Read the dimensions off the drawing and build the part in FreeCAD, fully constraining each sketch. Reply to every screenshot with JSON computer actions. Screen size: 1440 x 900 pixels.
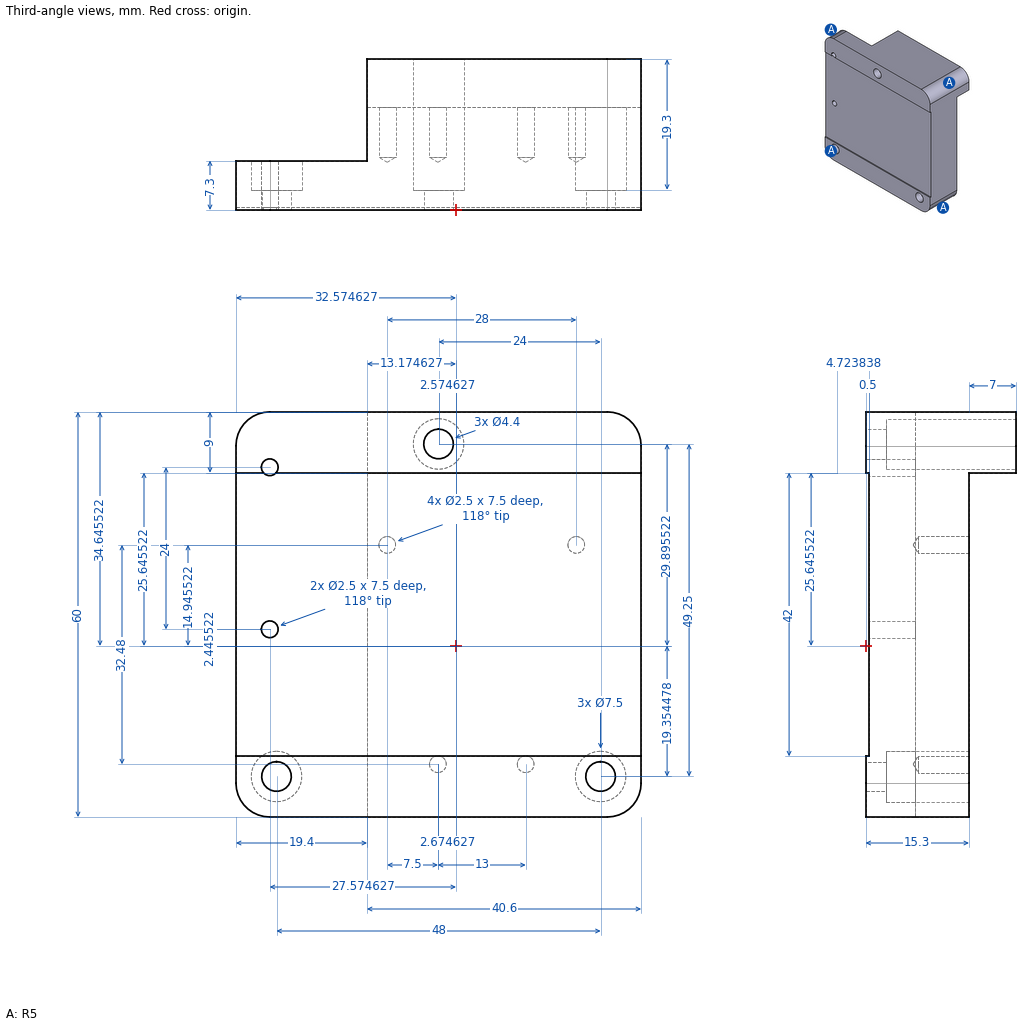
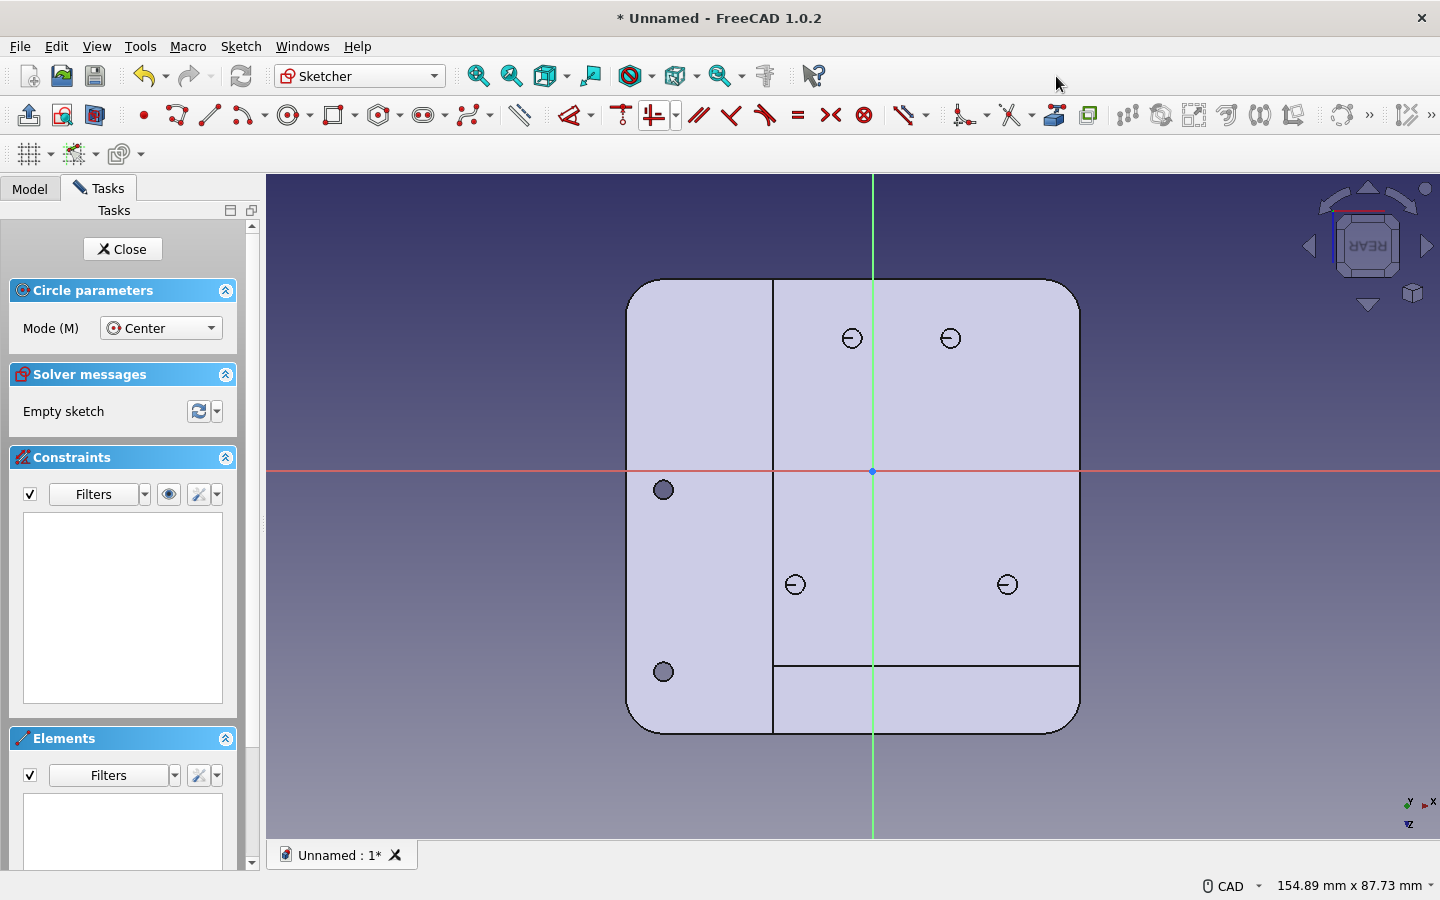
{"action": "left_click", "coordinate": [1035, 325]}
{"action": "left_click", "coordinate": [1055, 304]}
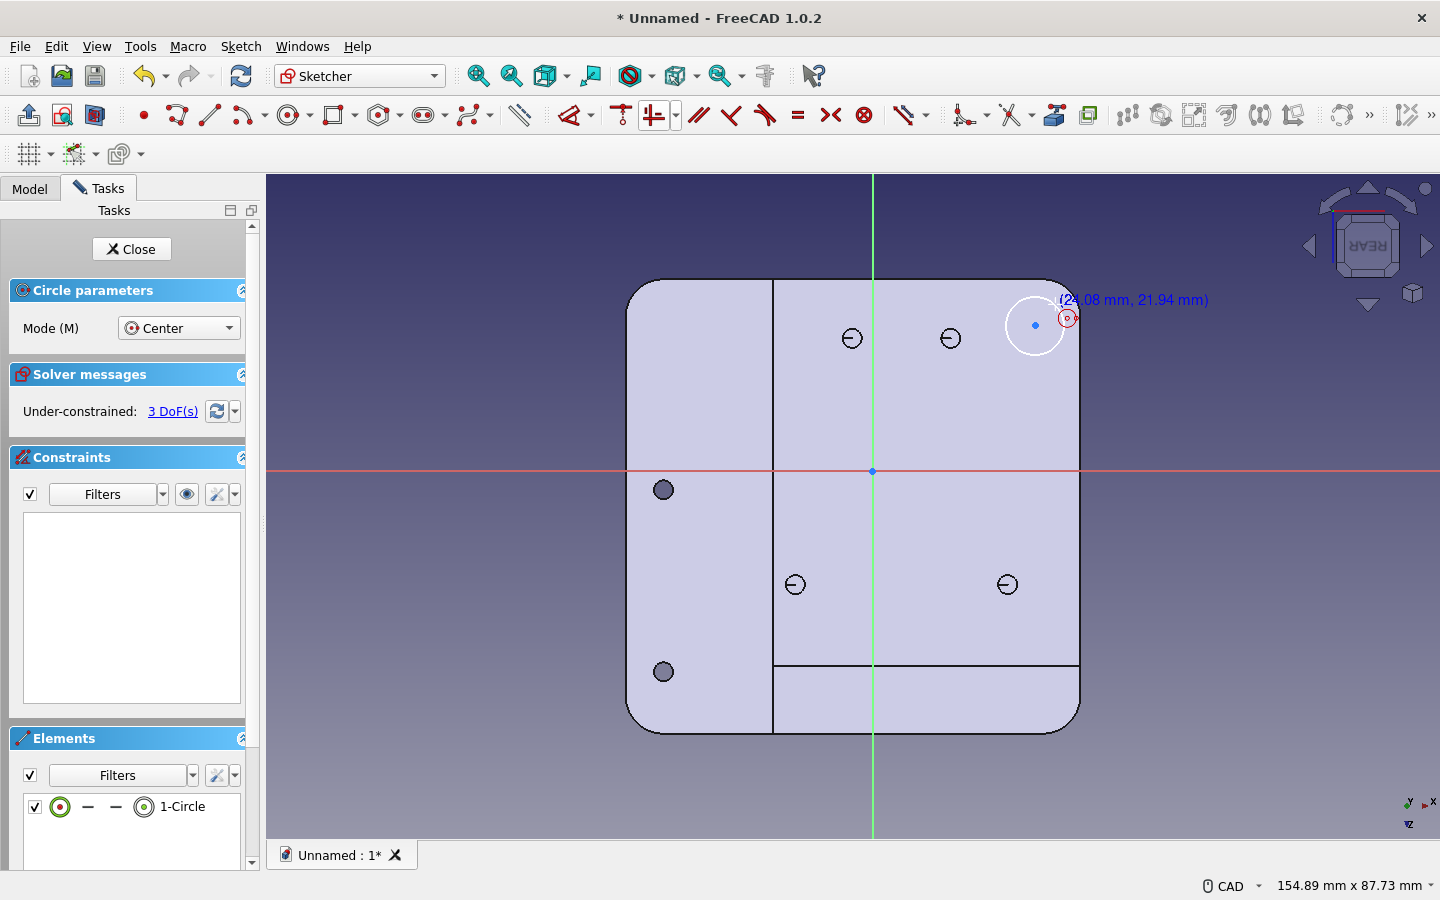
{"action": "left_click", "coordinate": [671, 325]}
{"action": "left_click", "coordinate": [691, 304]}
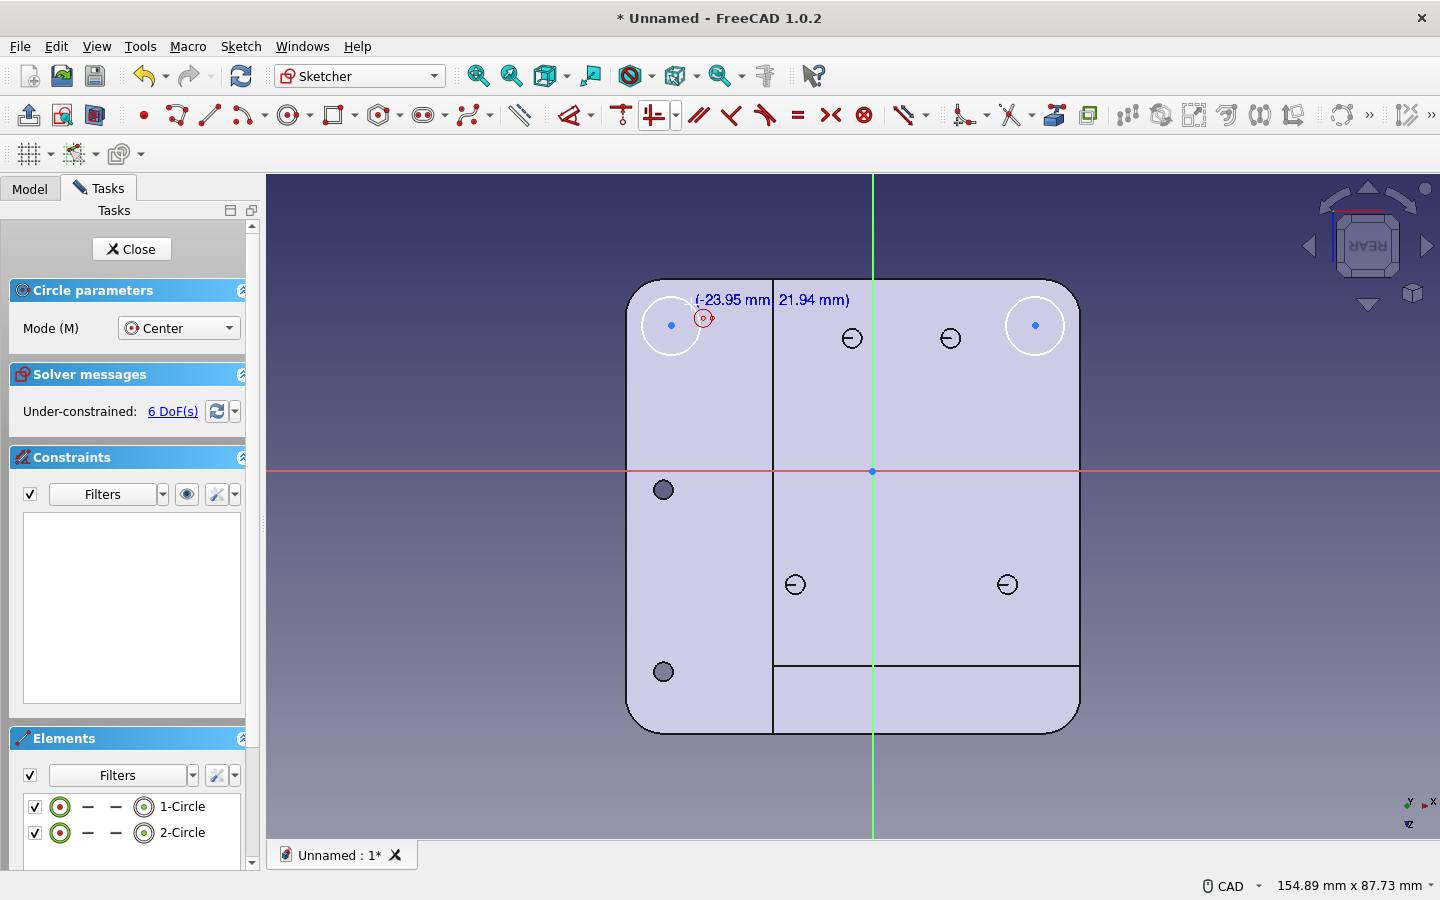
{"action": "left_click", "coordinate": [853, 698]}
{"action": "left_click", "coordinate": [833, 678]}
{"action": "key", "text": "Escape"}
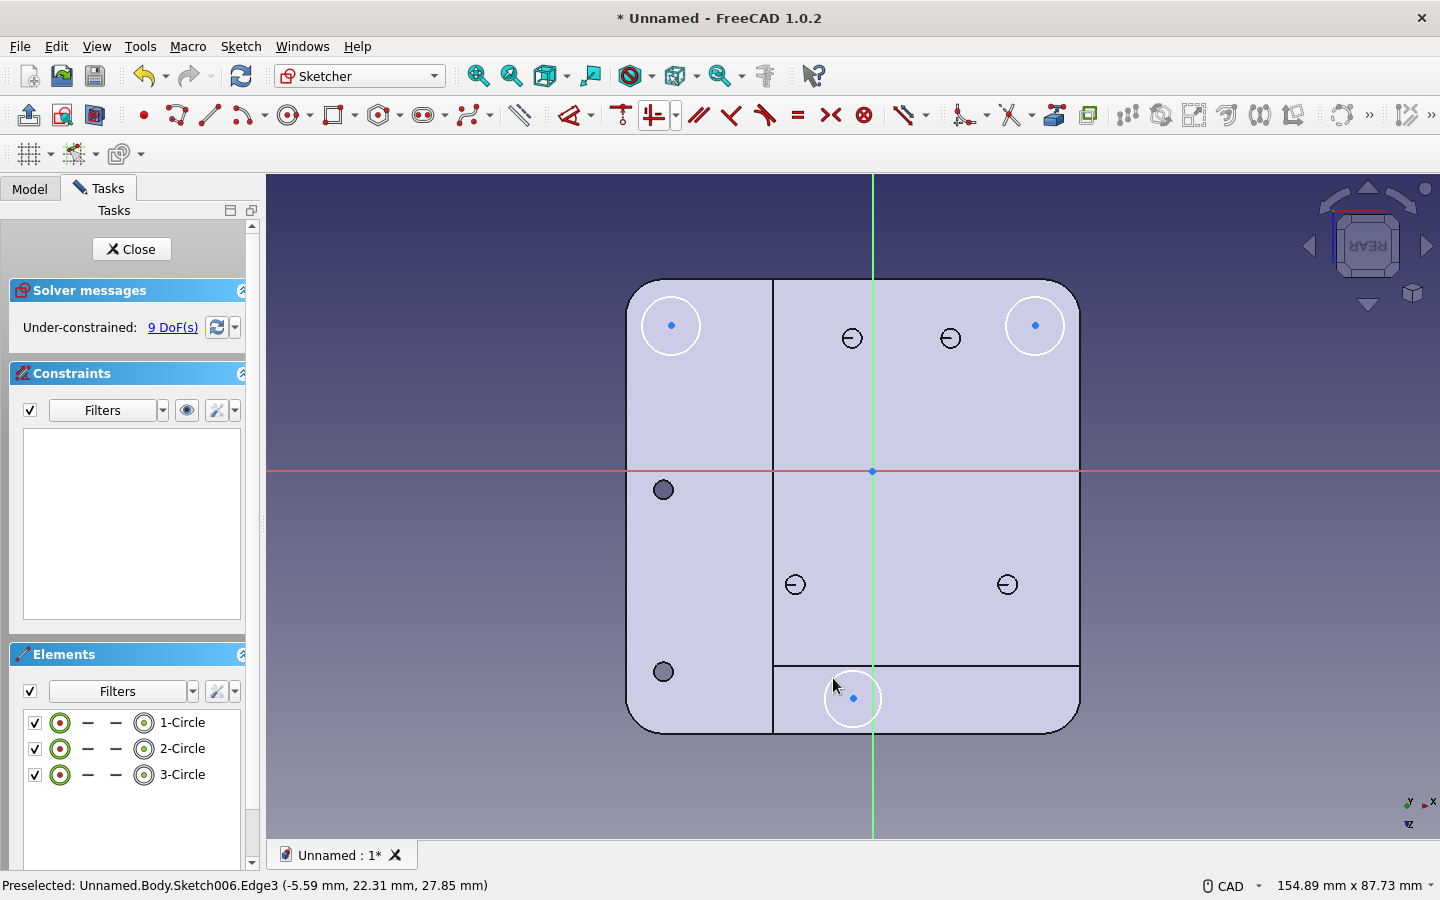
{"action": "left_click", "coordinate": [1055, 305]}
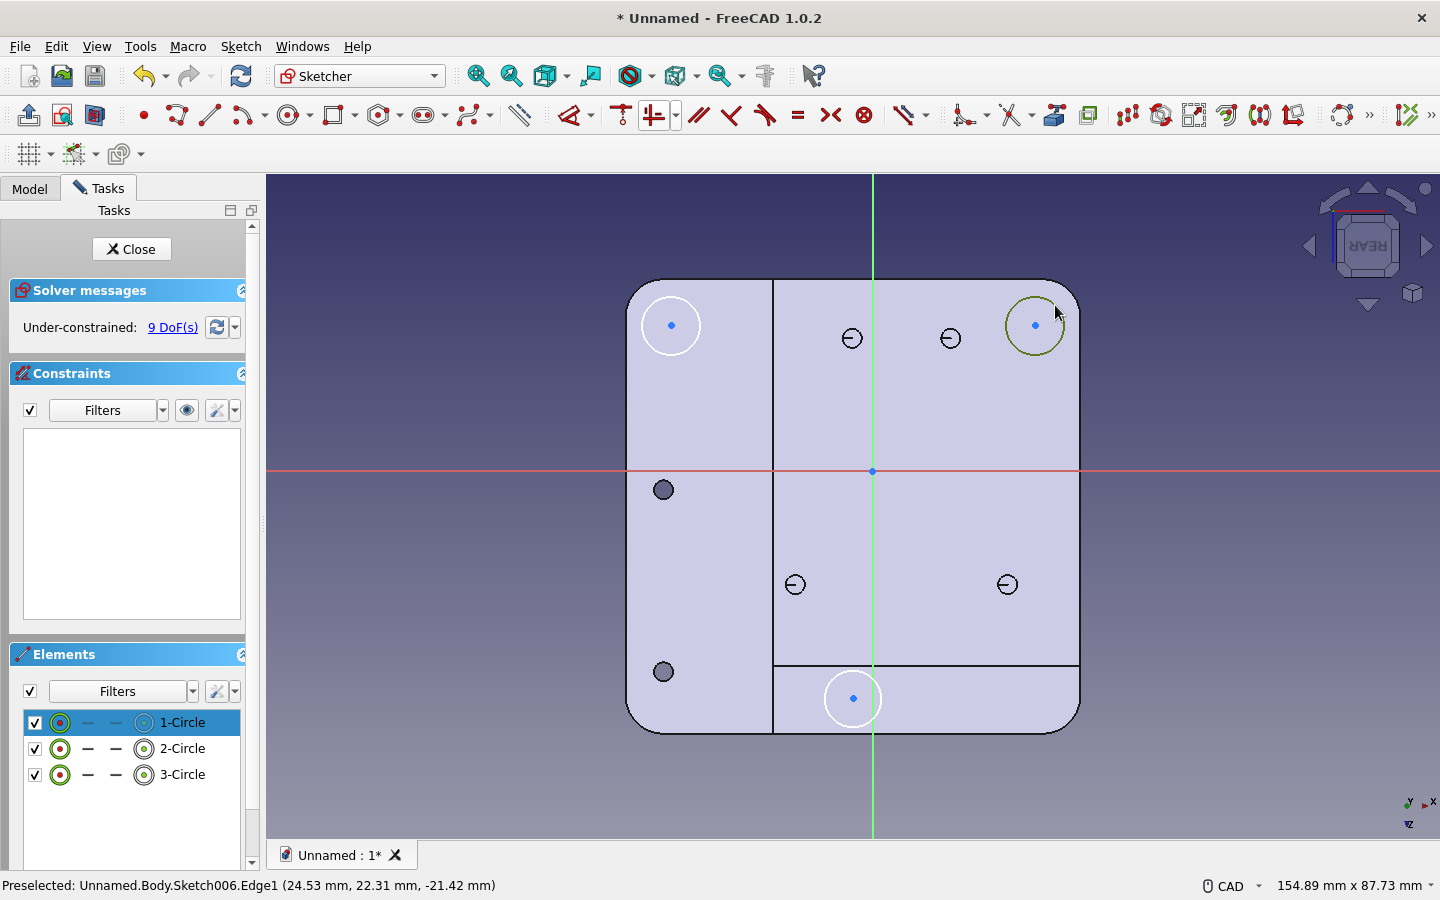
{"action": "left_click", "coordinate": [691, 305]}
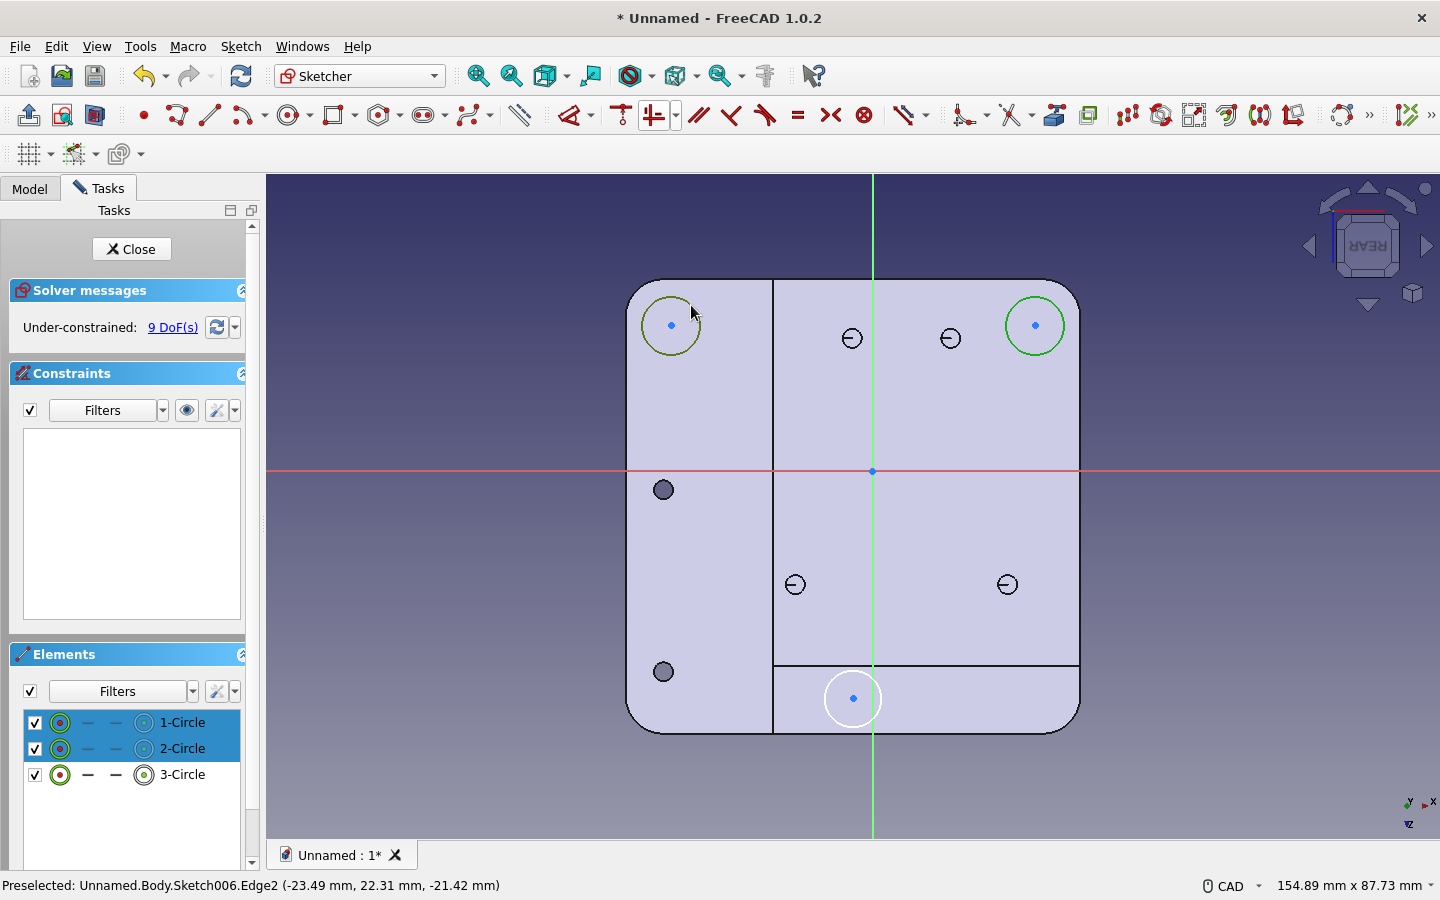
{"action": "left_click", "coordinate": [873, 679]}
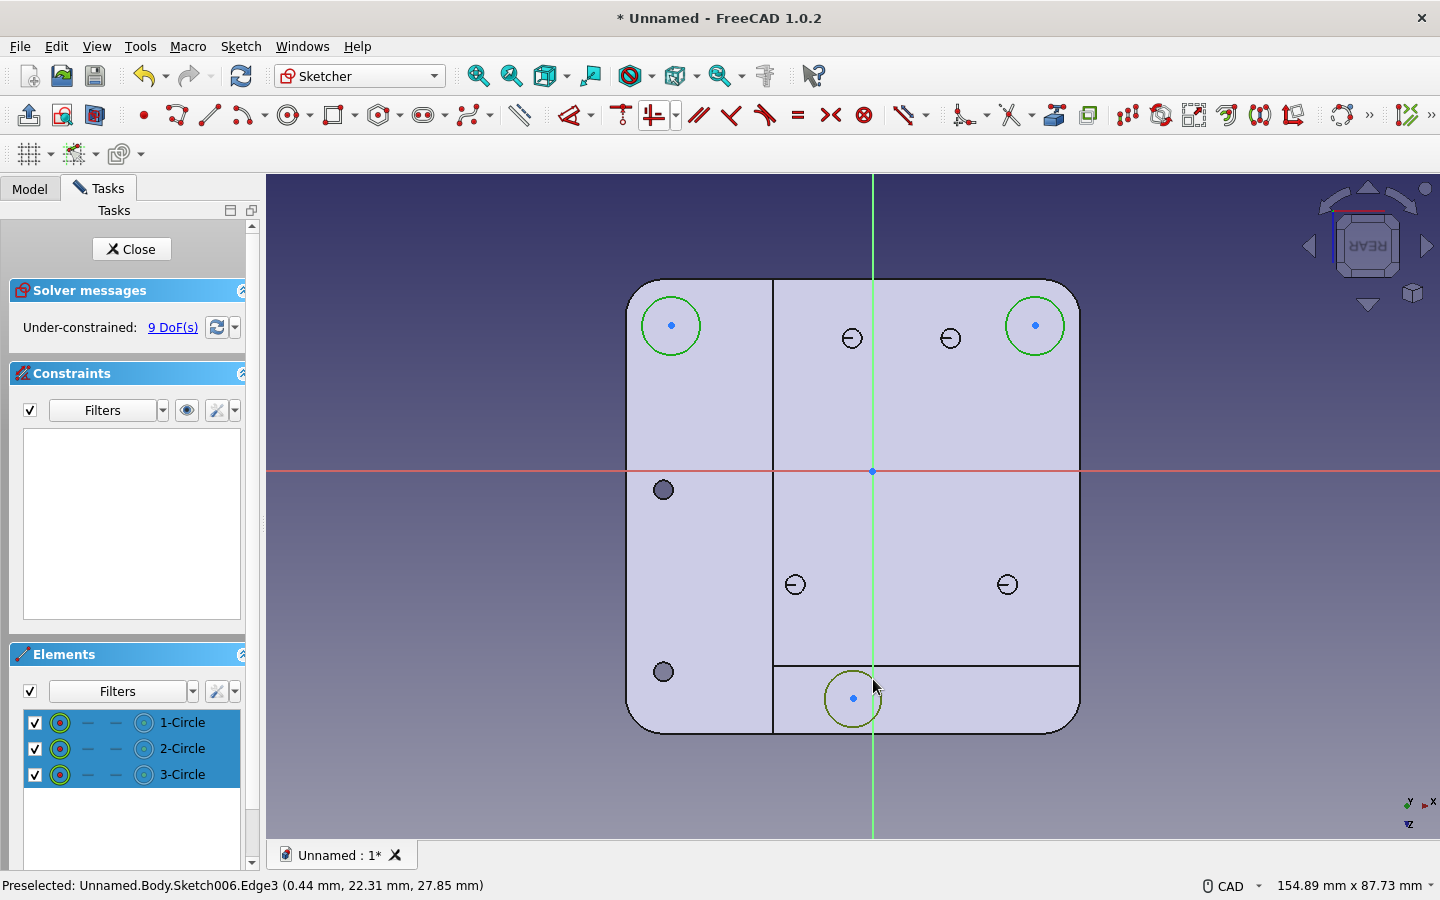
{"action": "left_click", "coordinate": [798, 116]}